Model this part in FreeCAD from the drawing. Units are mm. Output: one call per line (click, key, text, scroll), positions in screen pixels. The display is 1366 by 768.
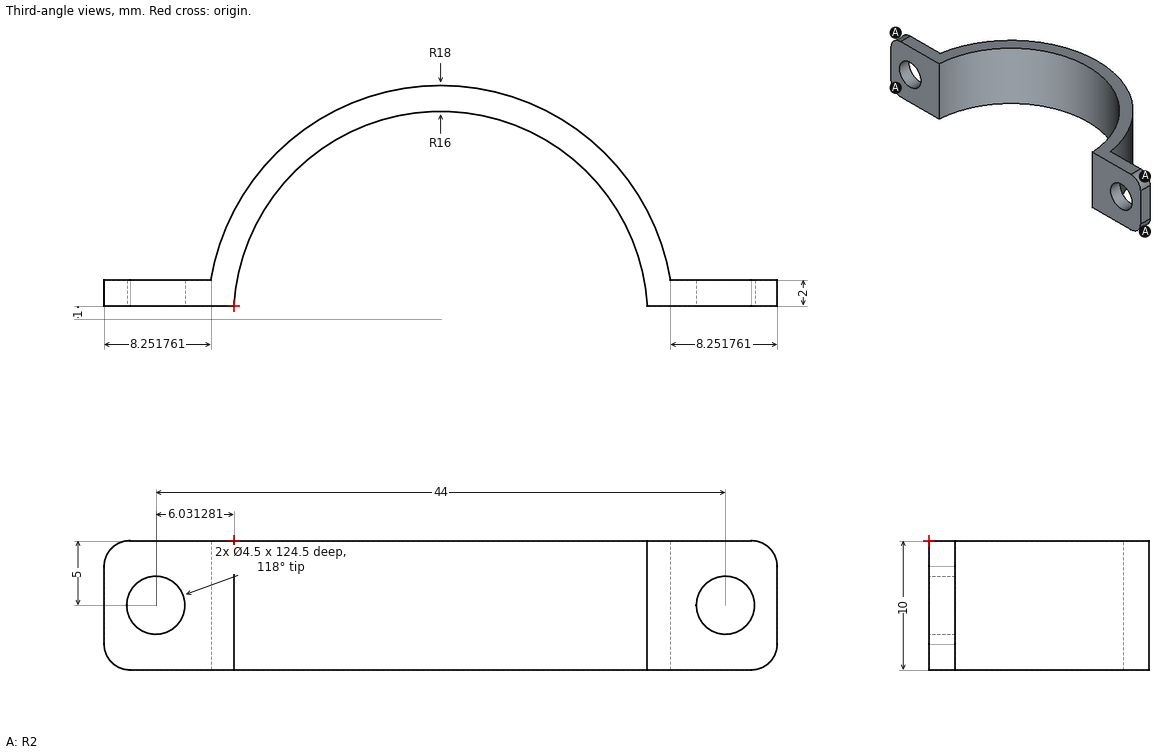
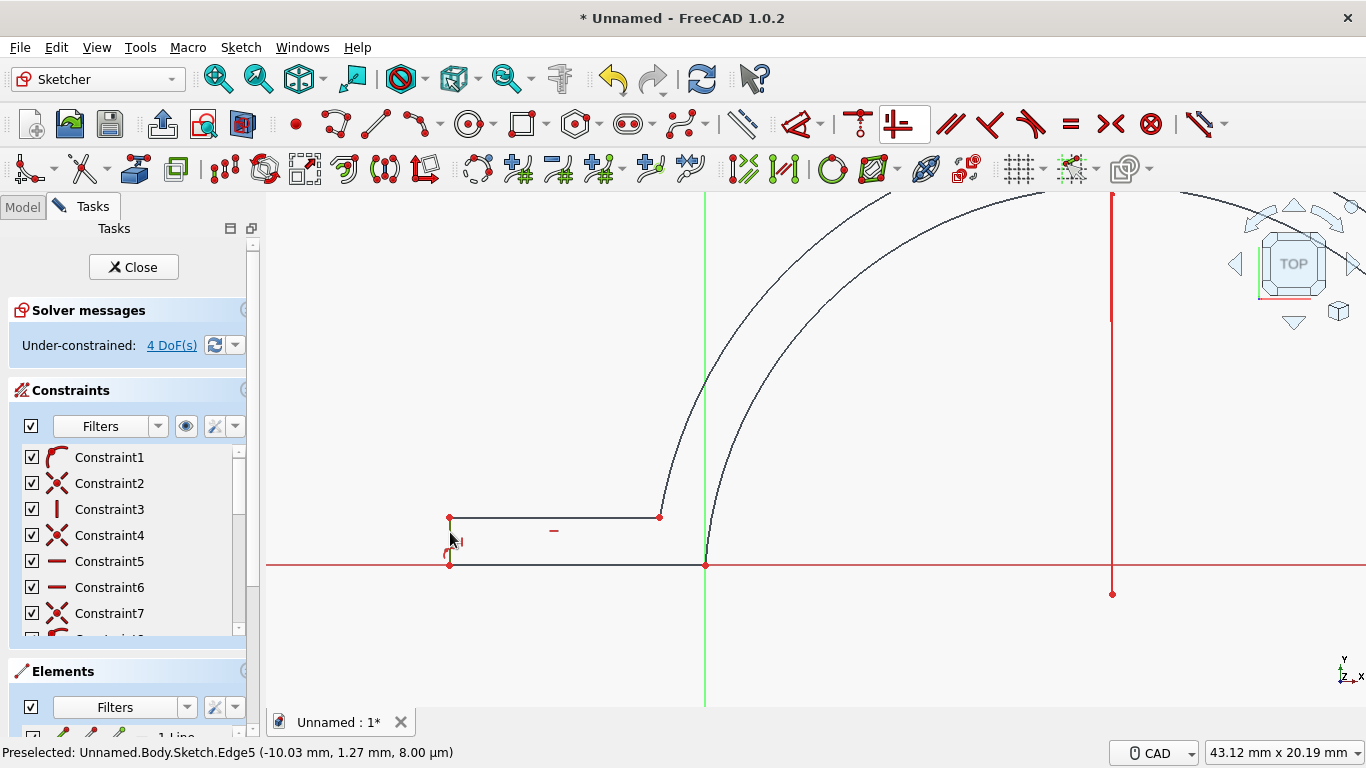
key(i)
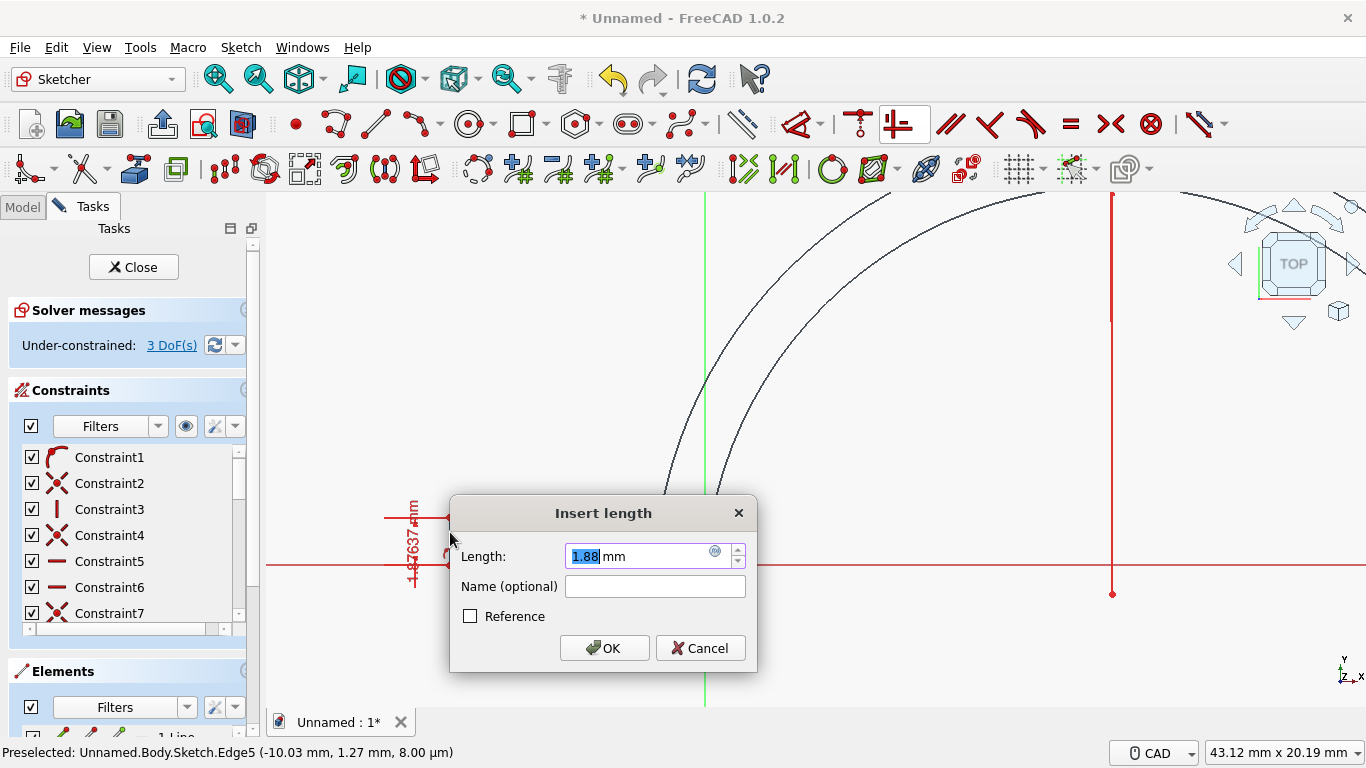
text(2)
key(Return)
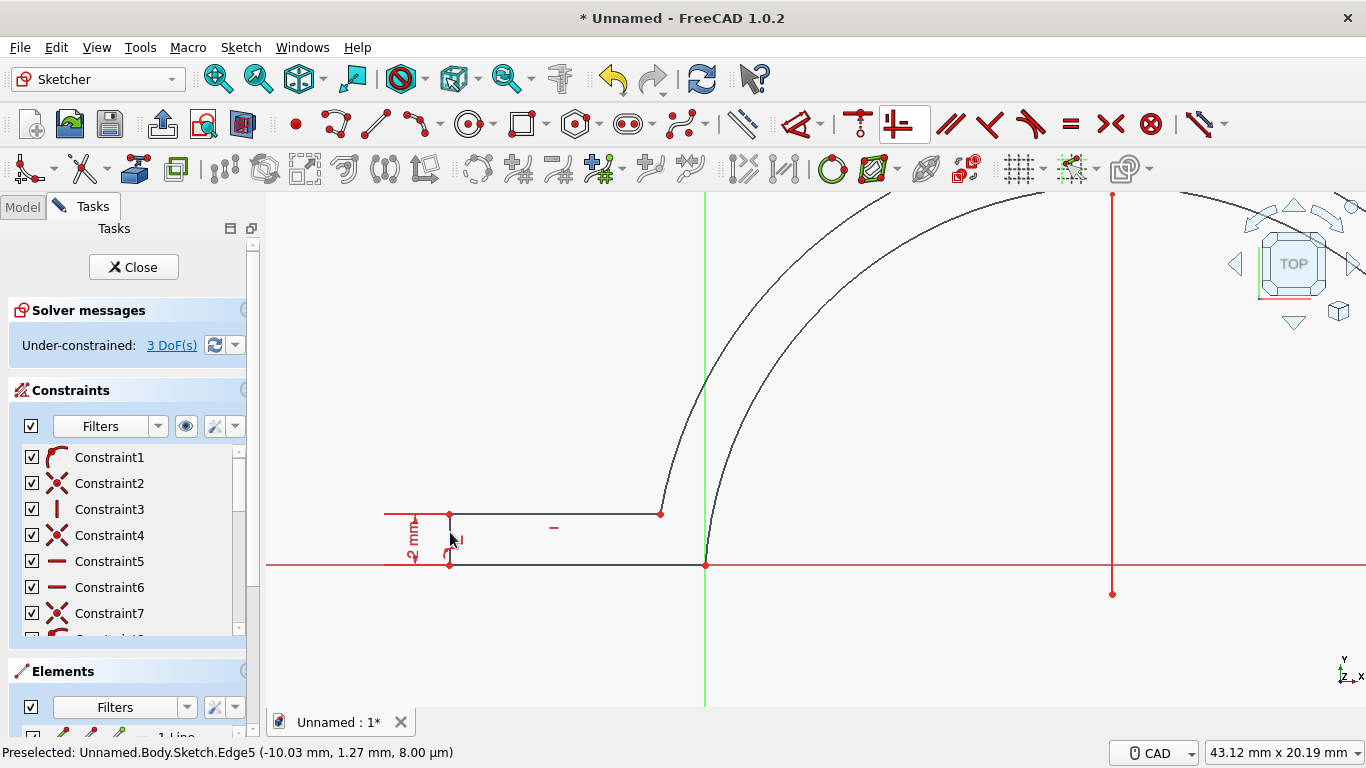
scroll(1112, 594, up, 3)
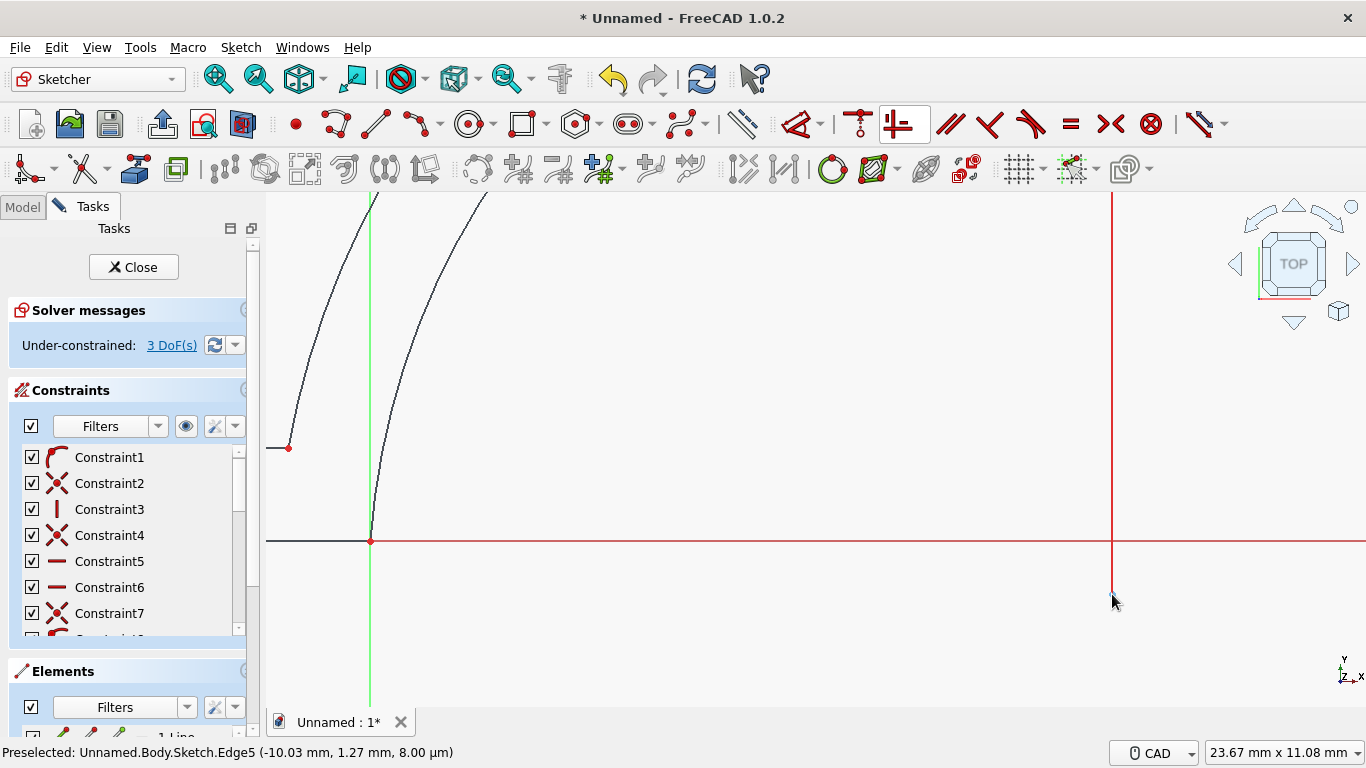
click(1112, 594)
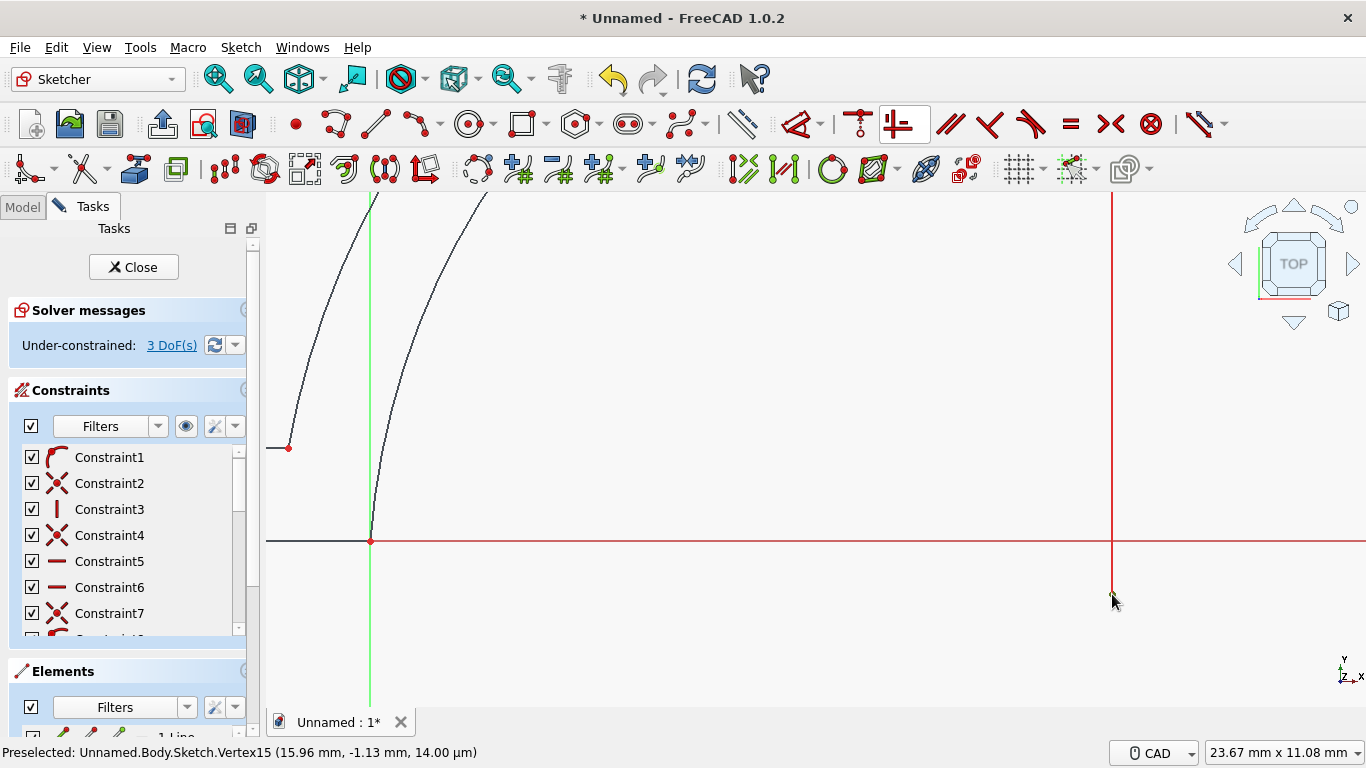
click(822, 124)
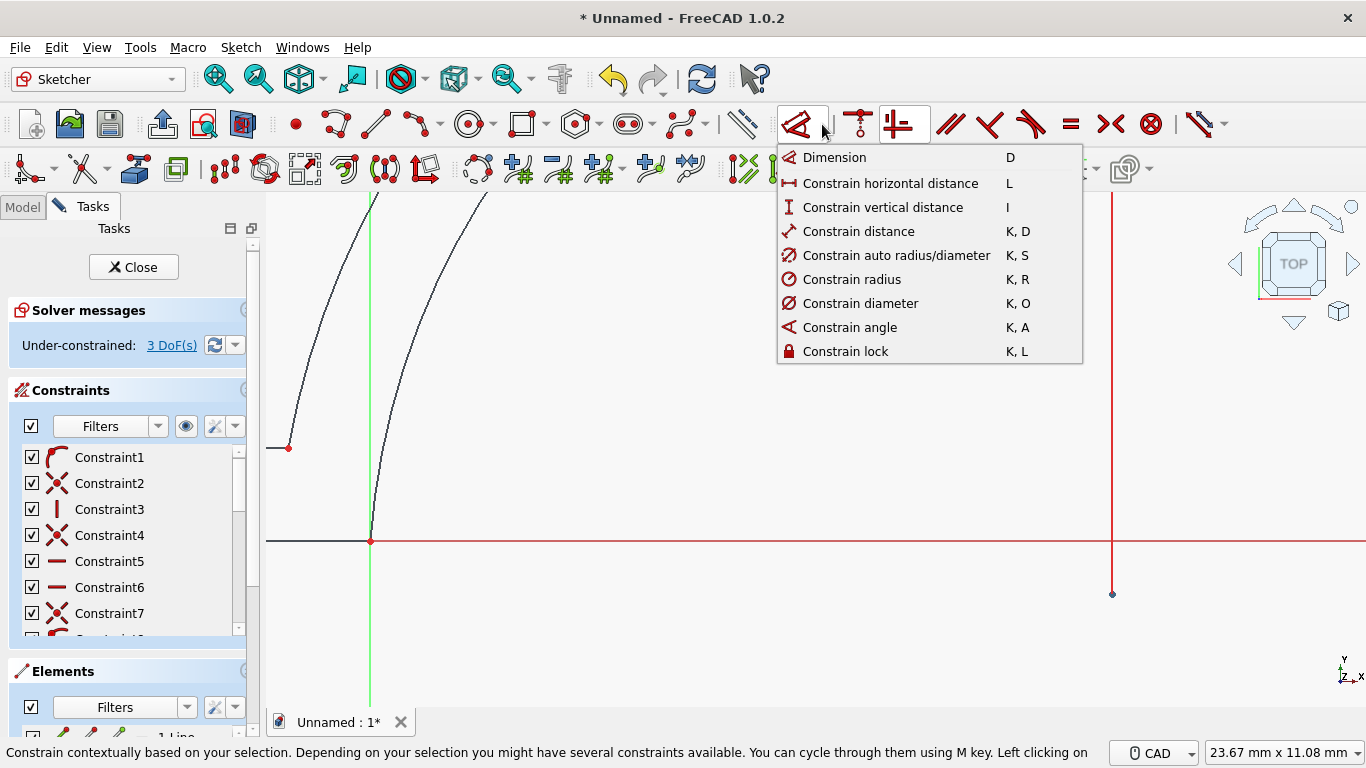
click(930, 207)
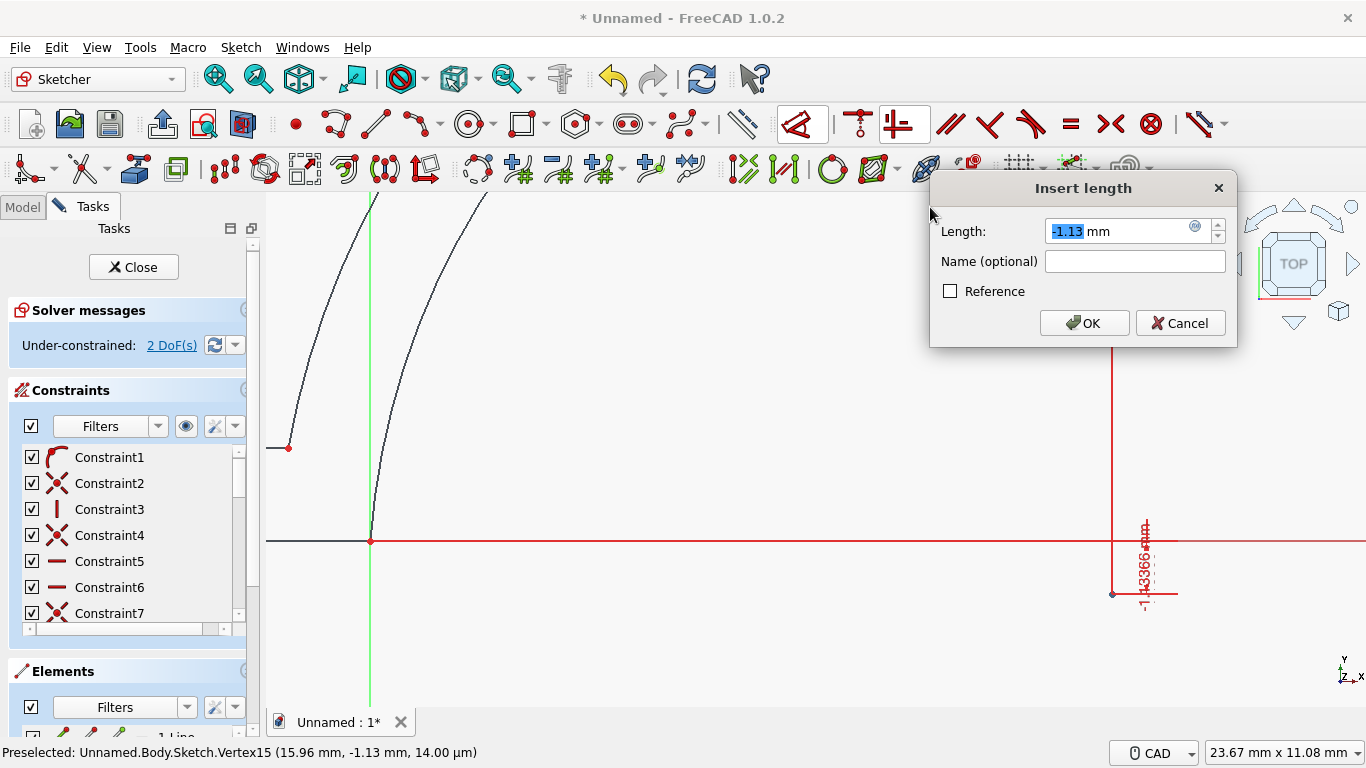
text(-1)
key(Return)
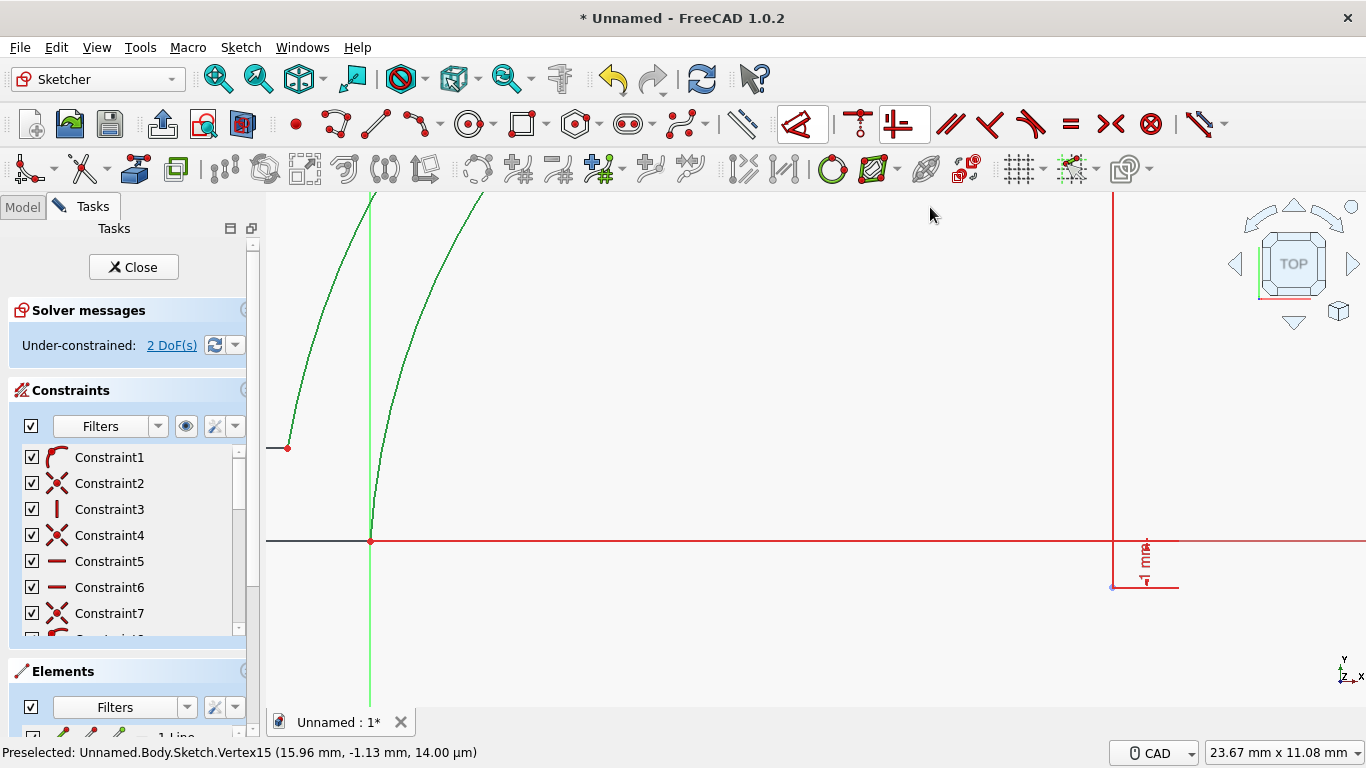
scroll(628, 549, down, 7)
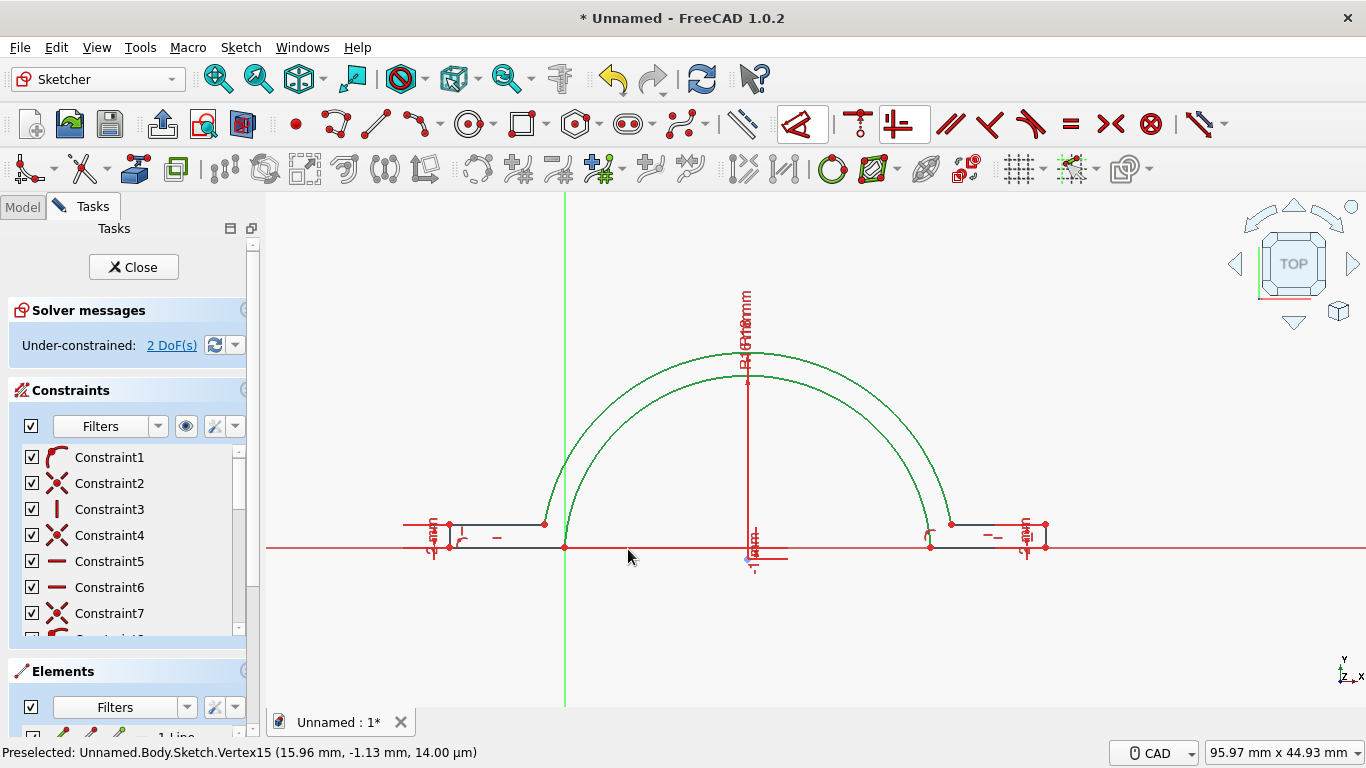
click(1017, 525)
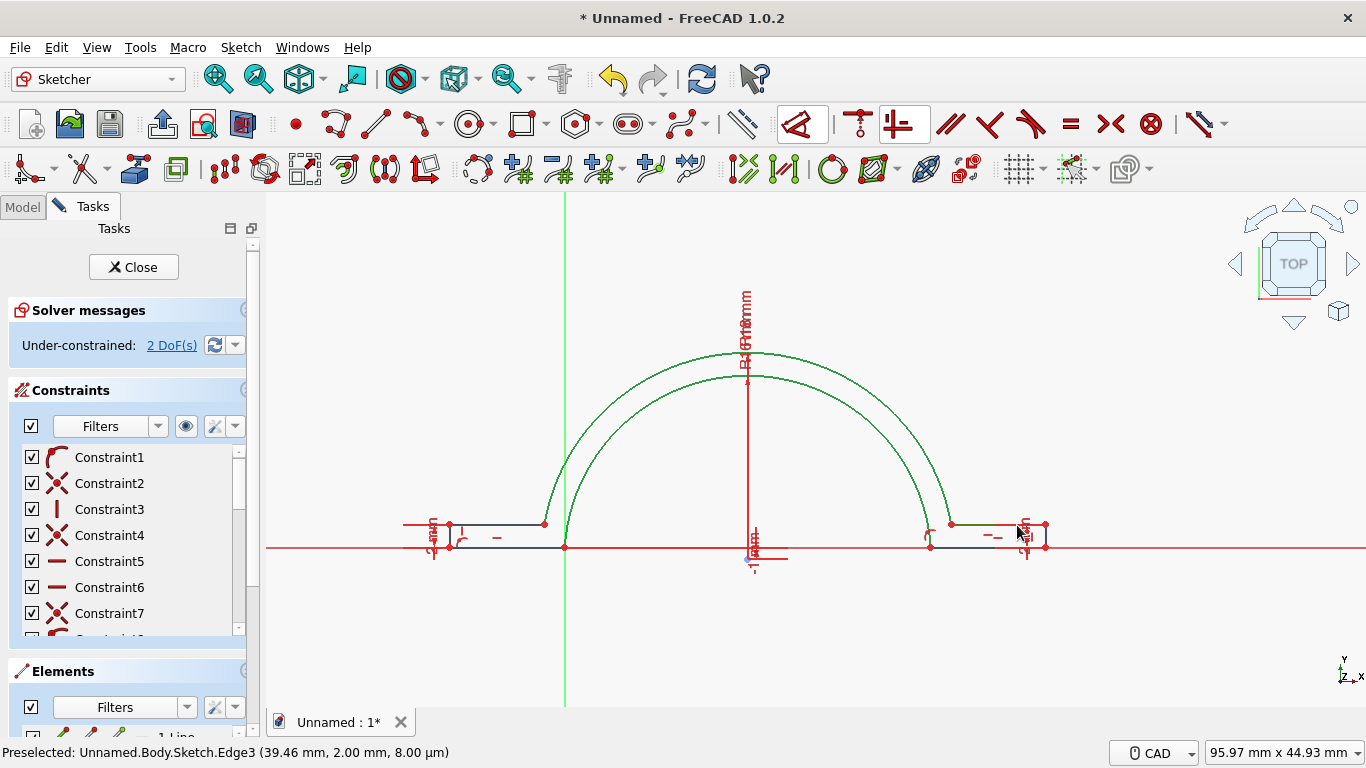
click(822, 124)